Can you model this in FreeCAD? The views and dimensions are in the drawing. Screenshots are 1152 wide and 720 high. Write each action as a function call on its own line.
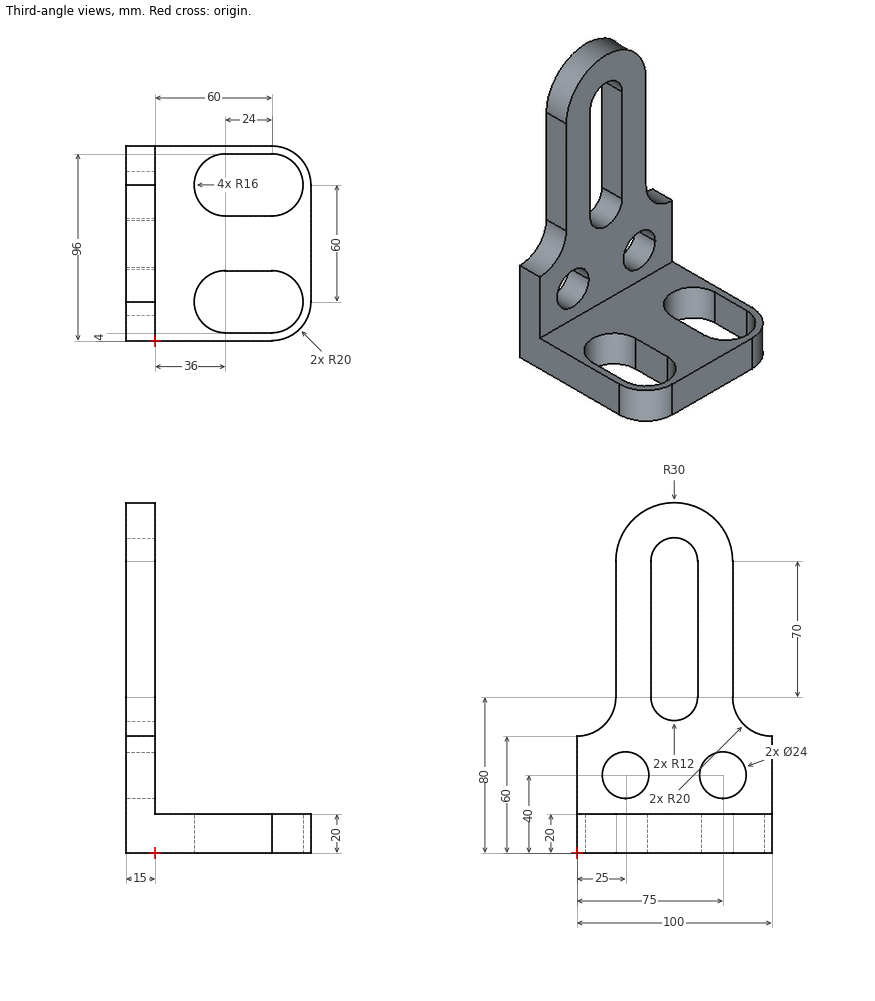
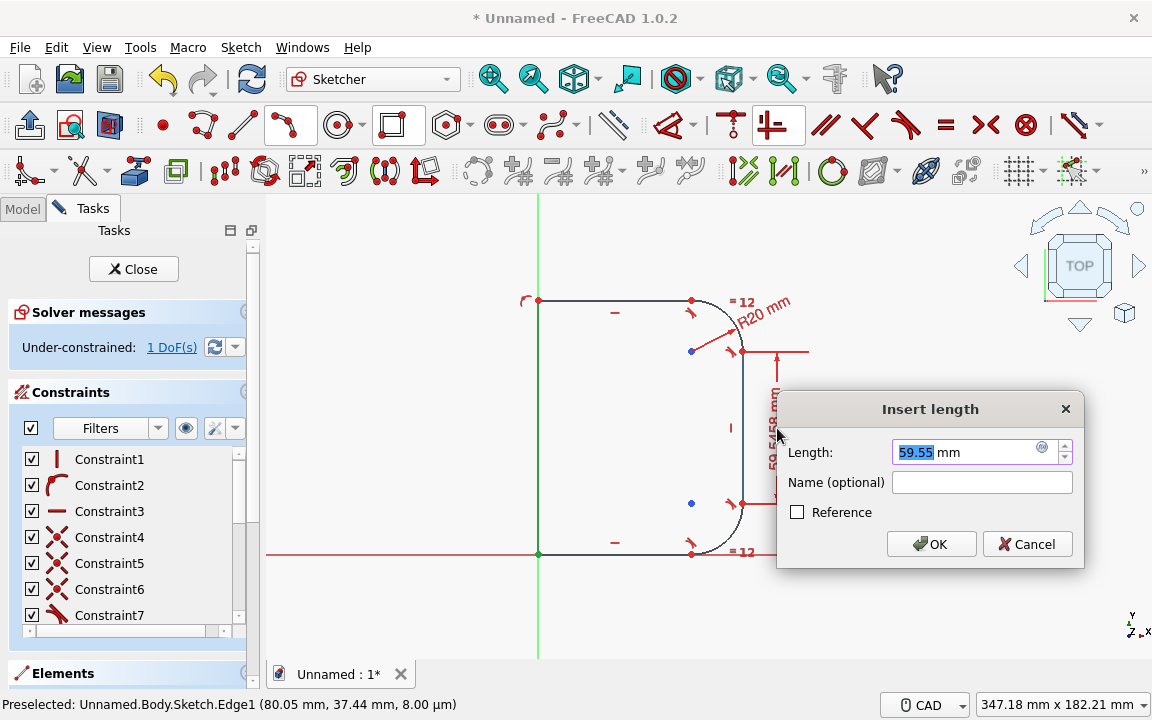
text(60)
key(Return)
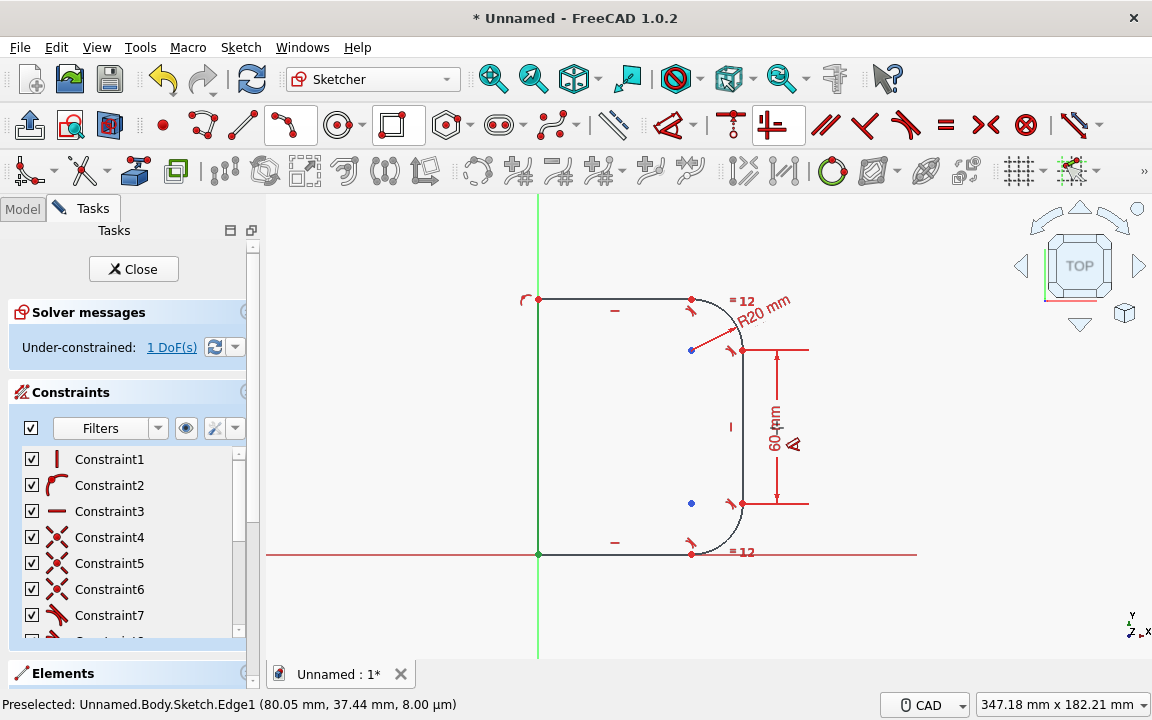
click(646, 299)
click(615, 265)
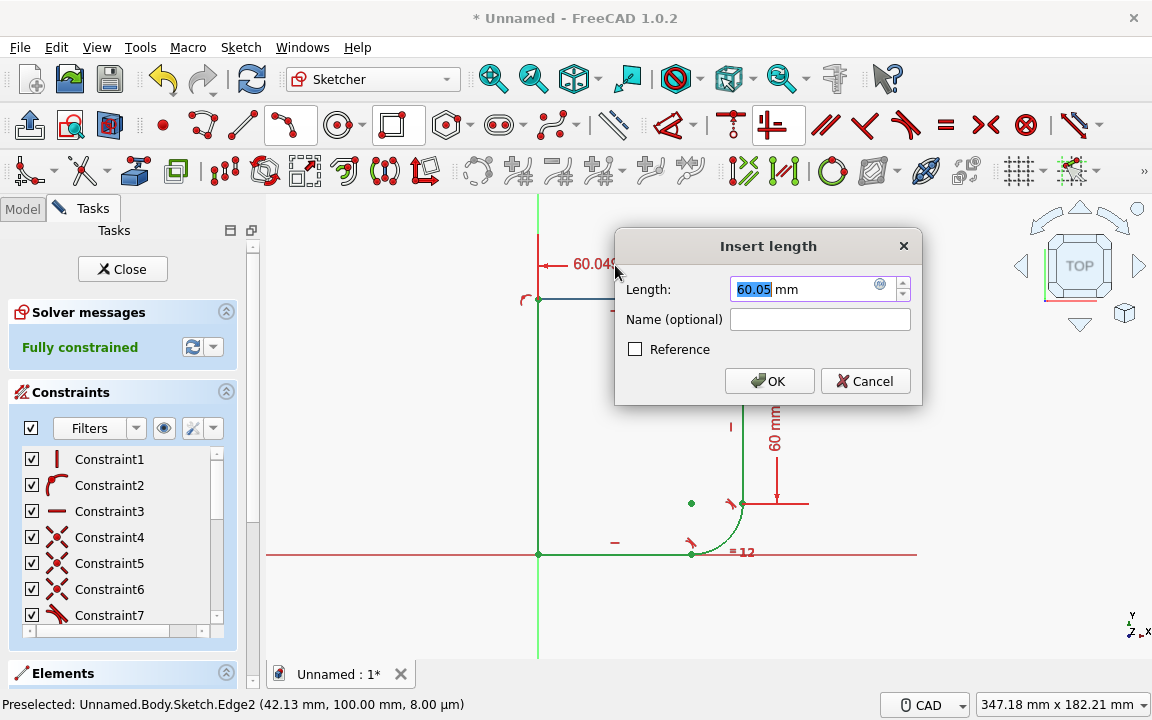
text(60)
key(Return)
key(Escape)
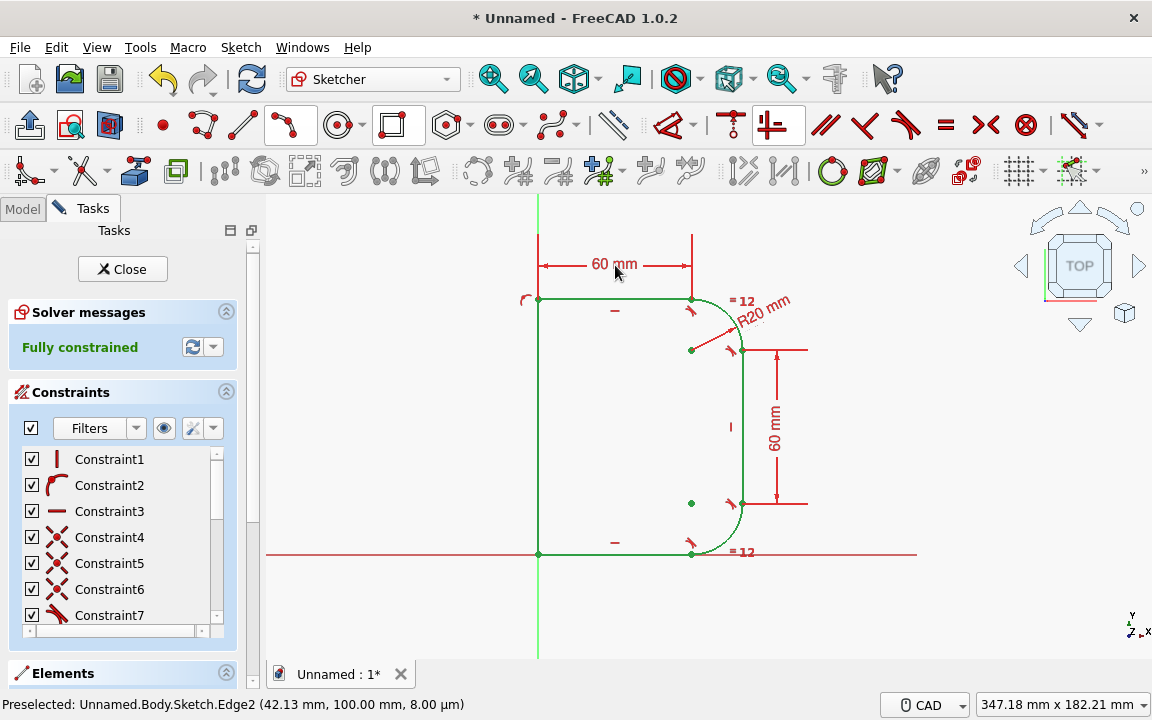
click(123, 269)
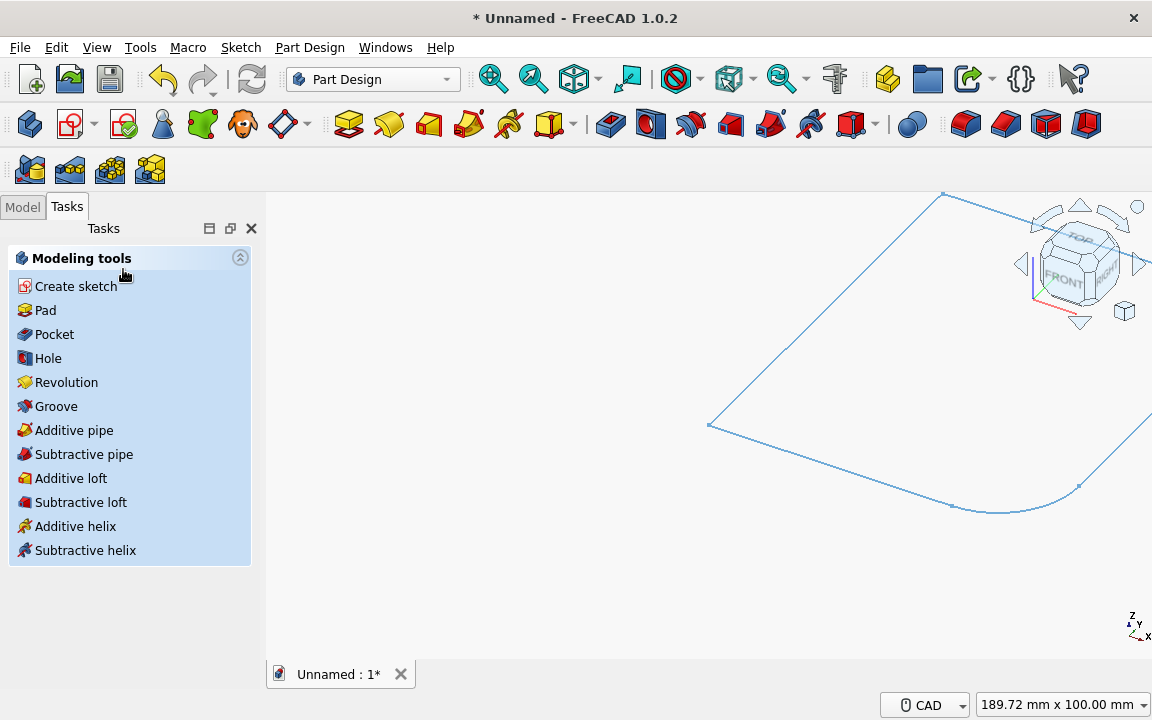
click(350, 124)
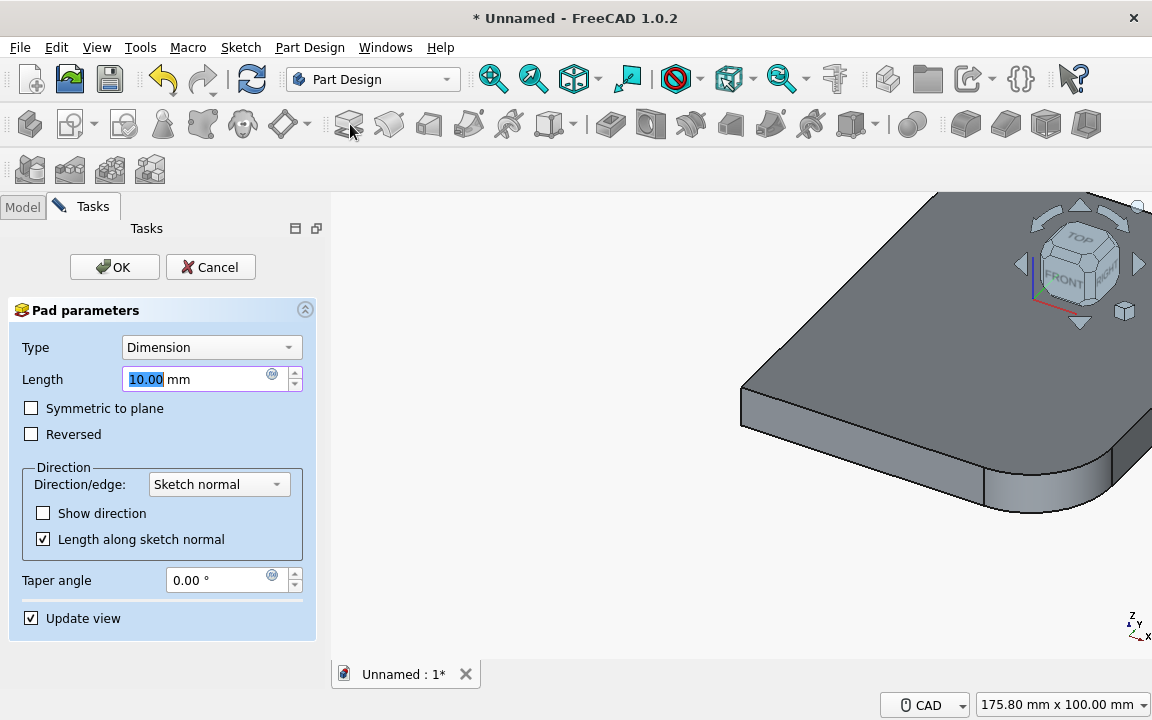
text(20)
key(Tab)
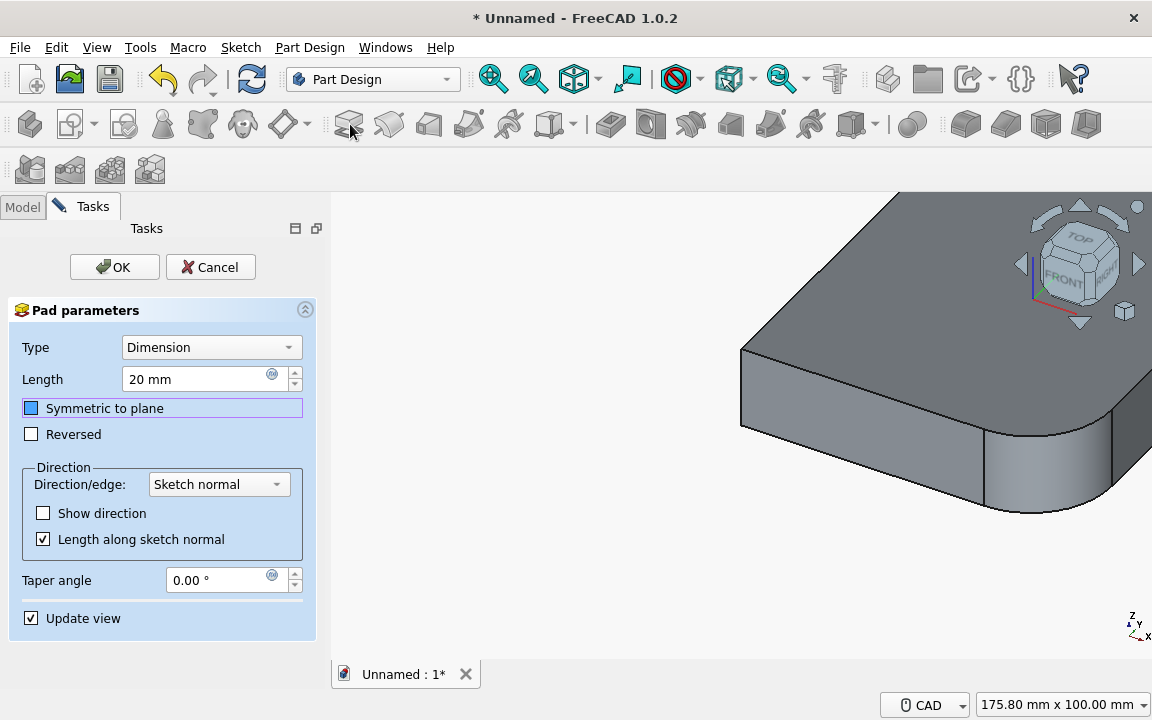
click(115, 267)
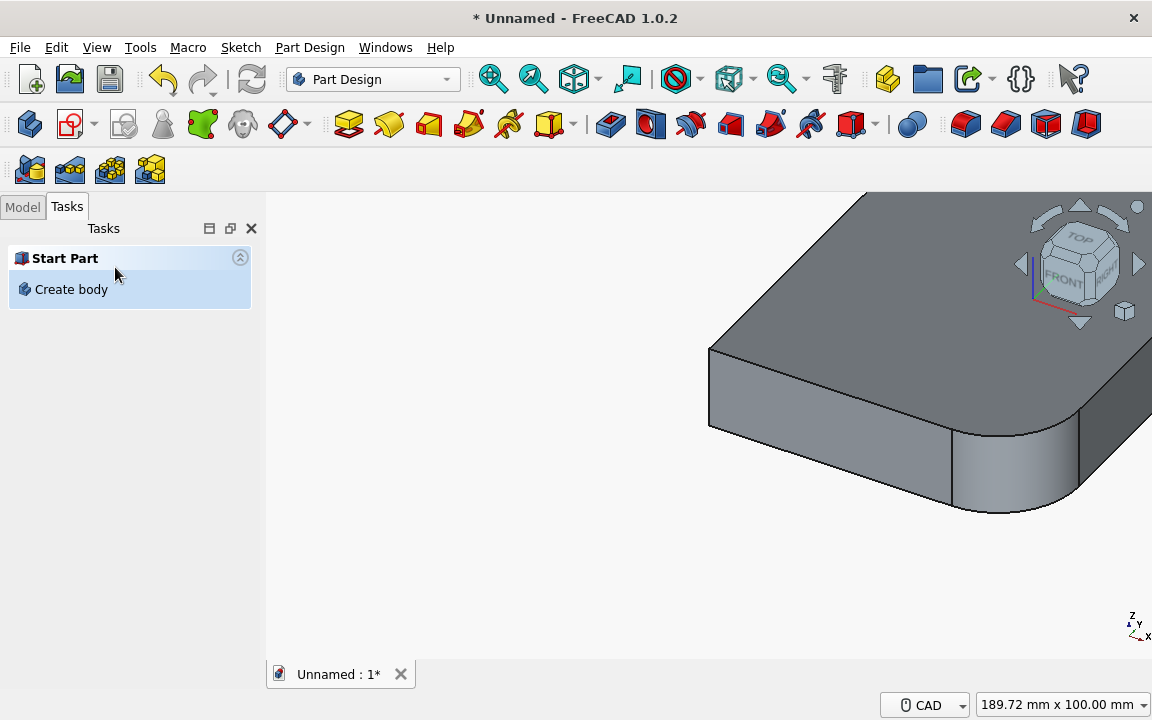
click(494, 80)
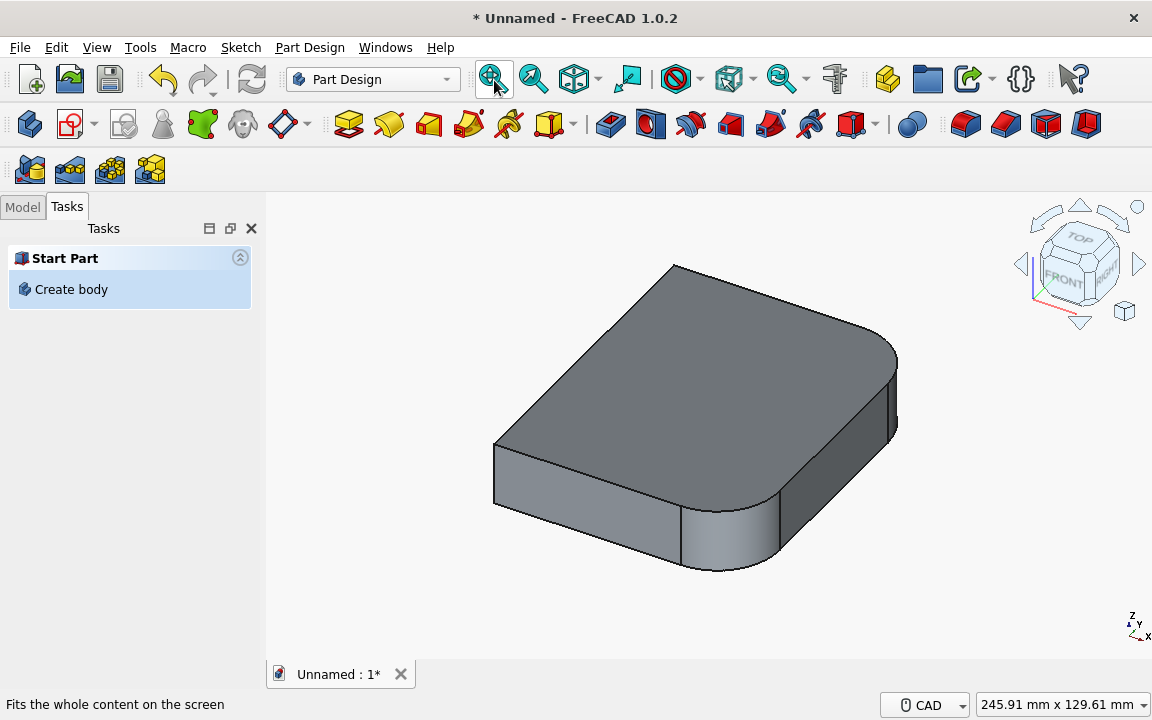
key(6)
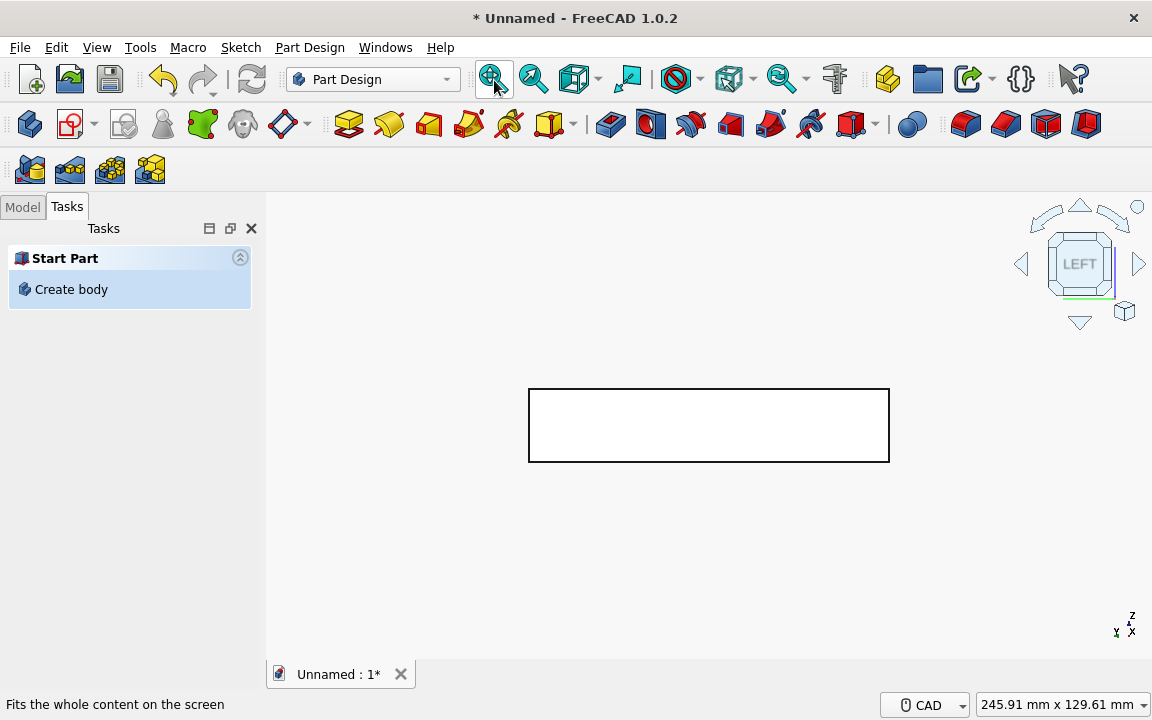
click(494, 80)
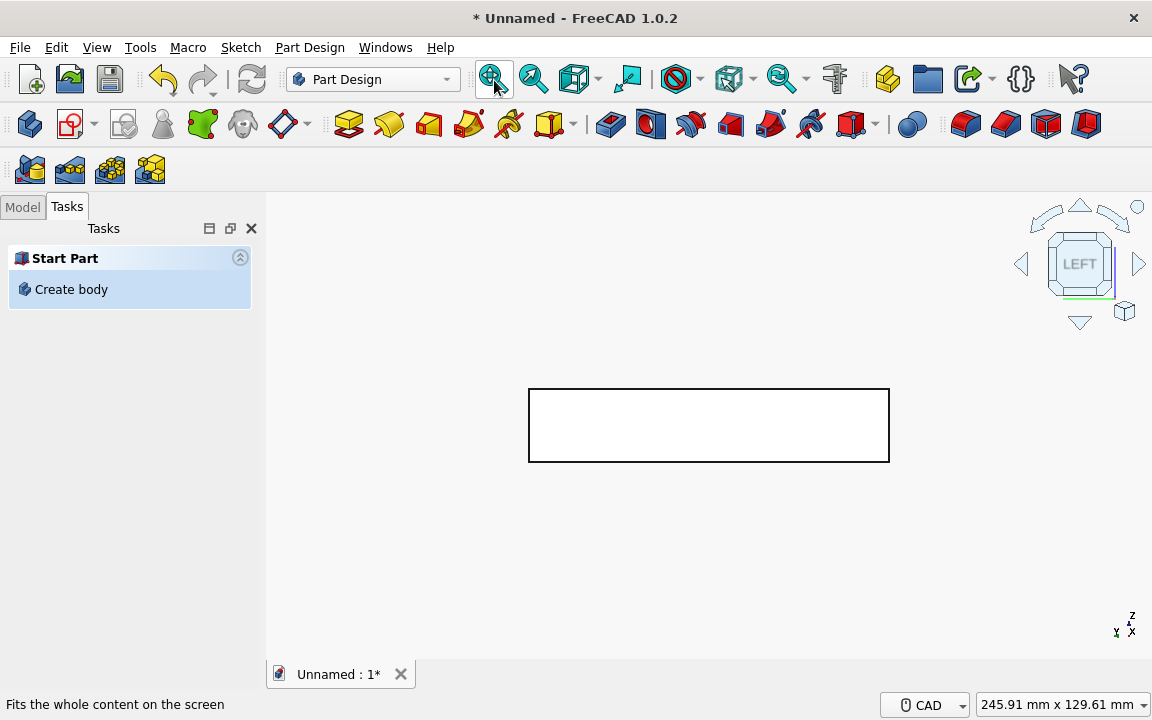
click(606, 424)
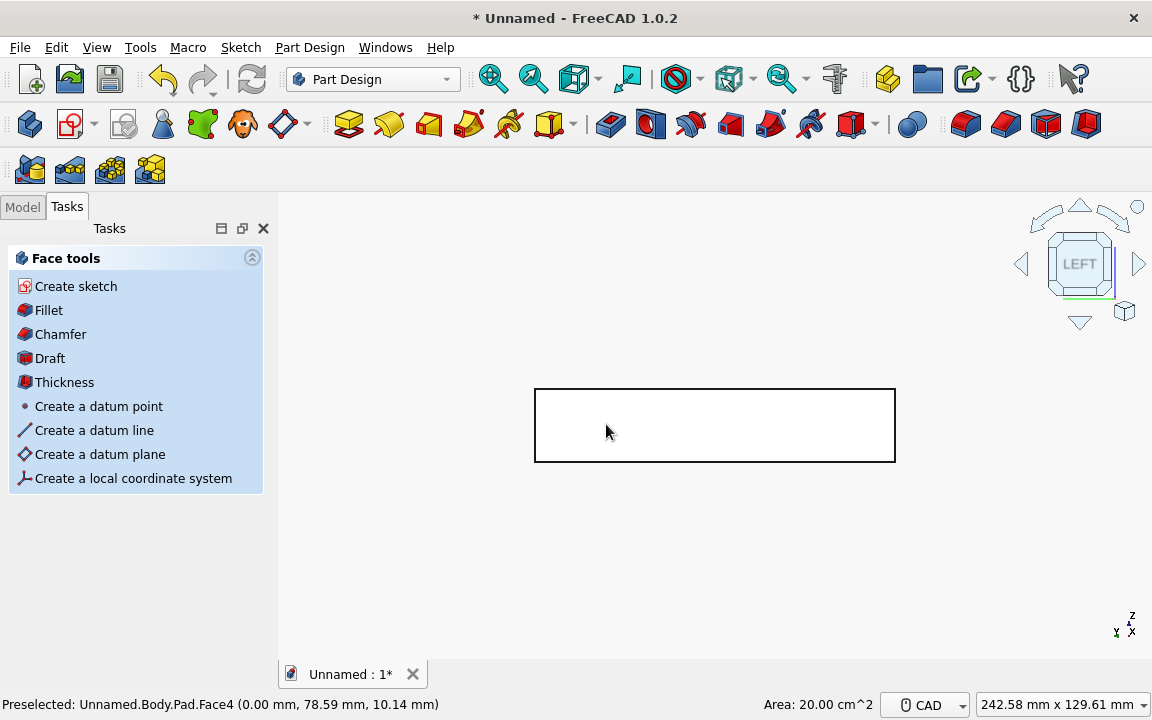
click(70, 124)